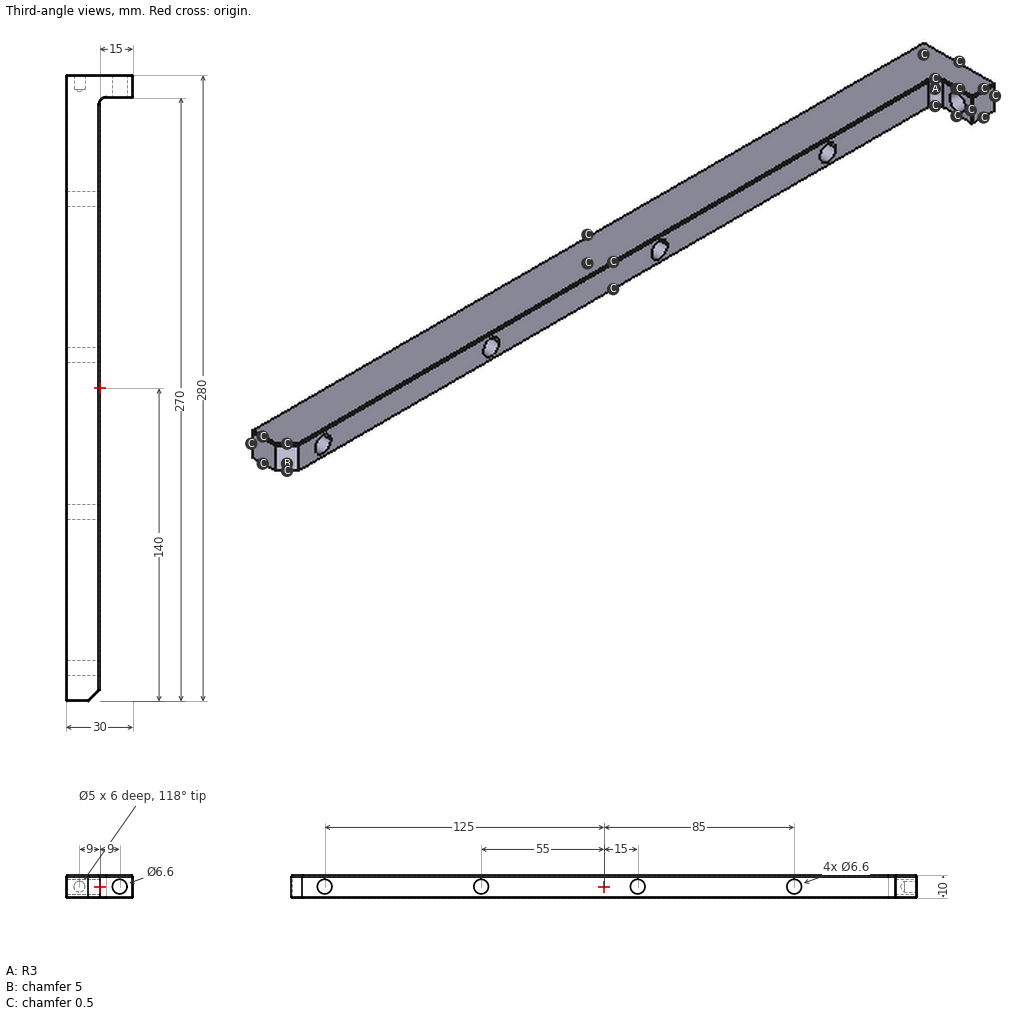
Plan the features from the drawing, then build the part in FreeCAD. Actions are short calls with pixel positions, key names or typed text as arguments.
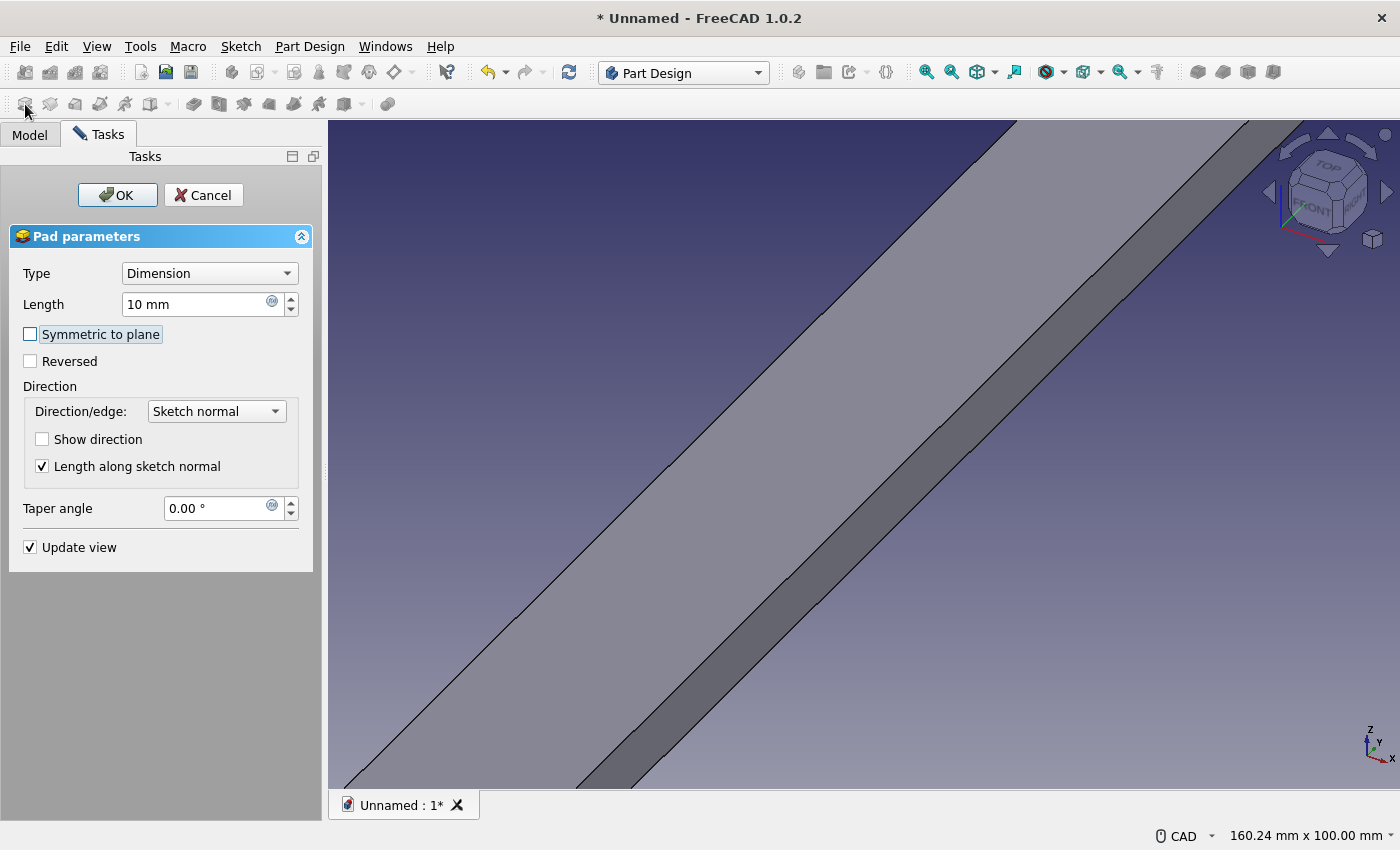
click(31, 334)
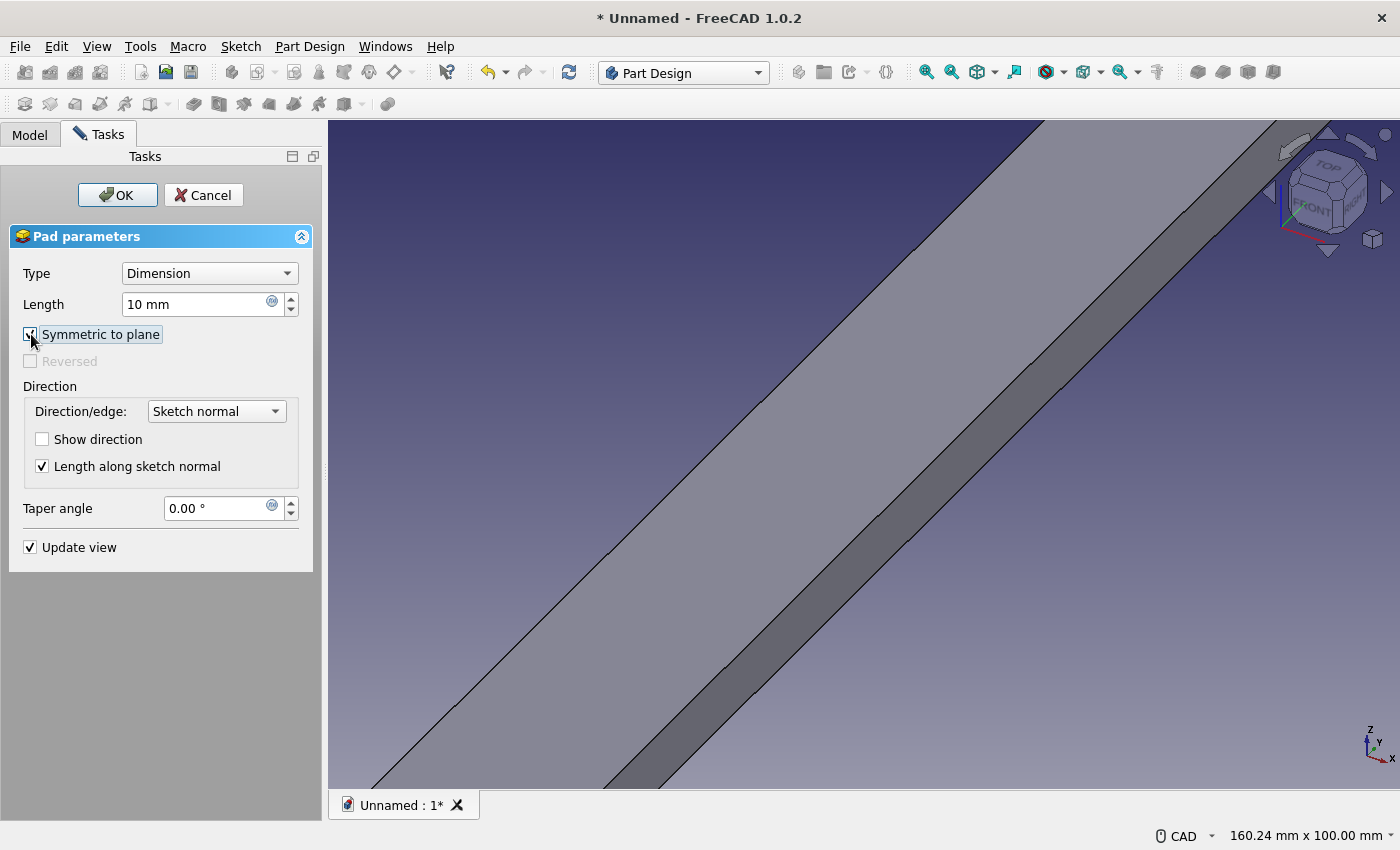
click(118, 195)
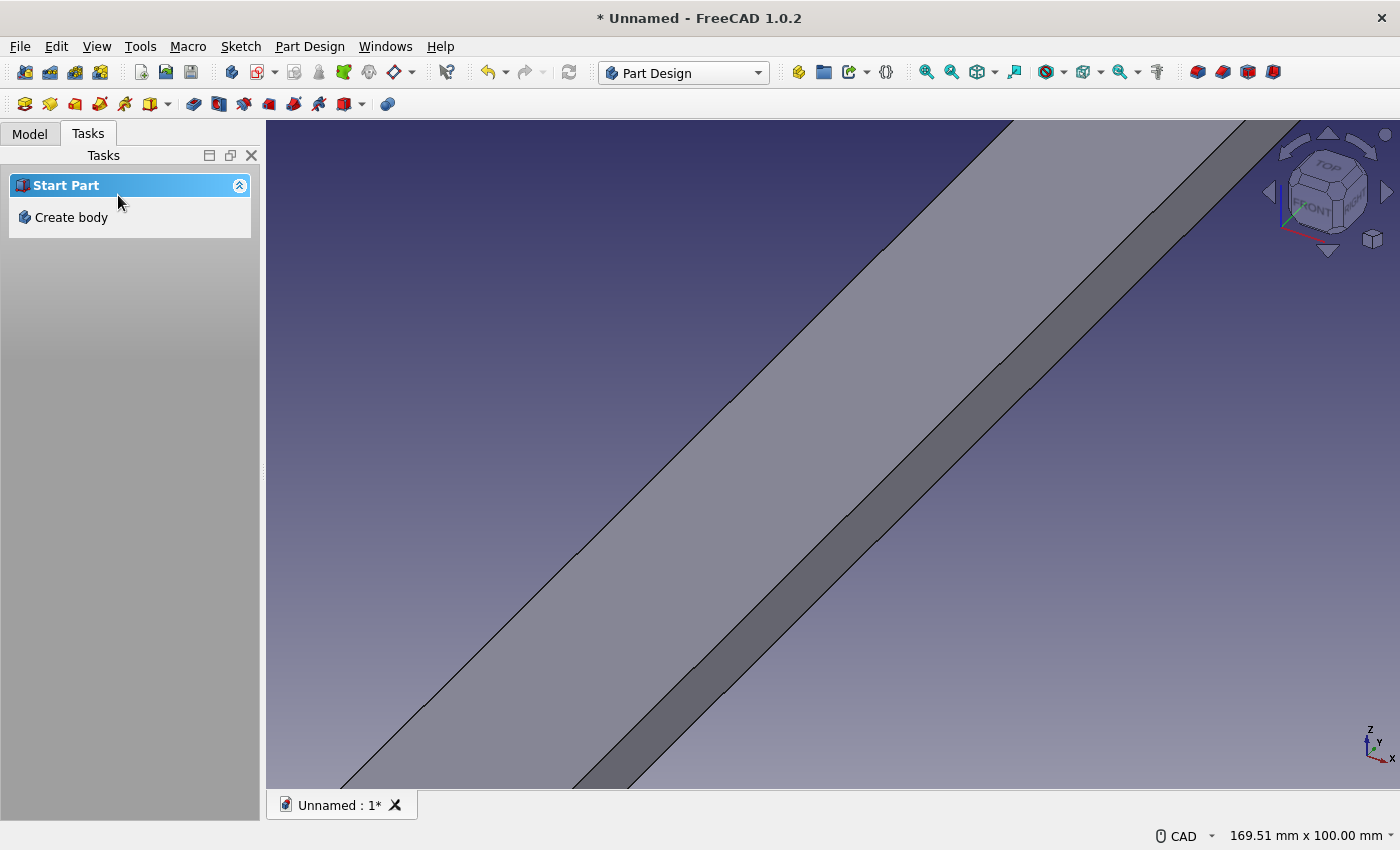
key(v)
key(f)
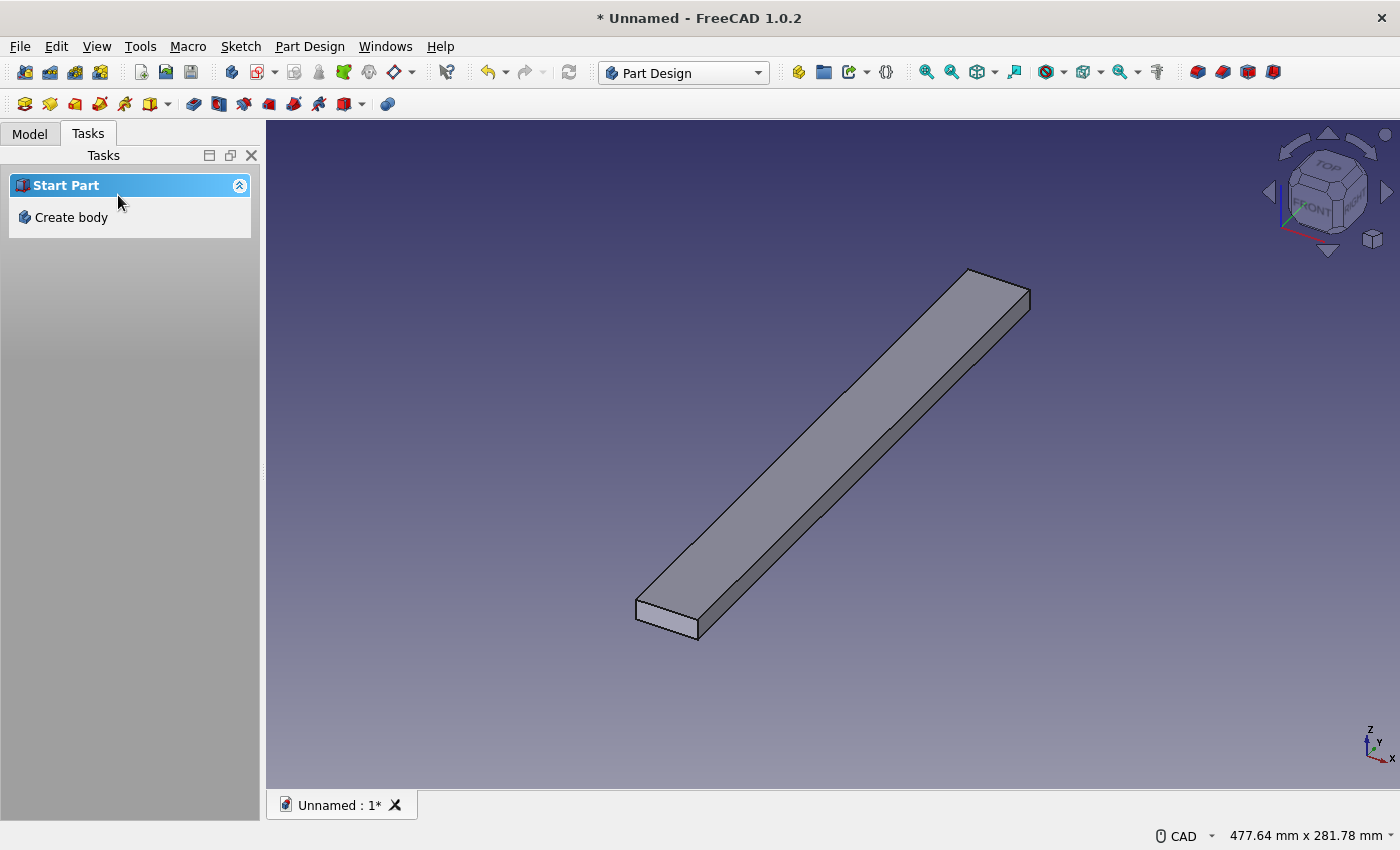
key(5)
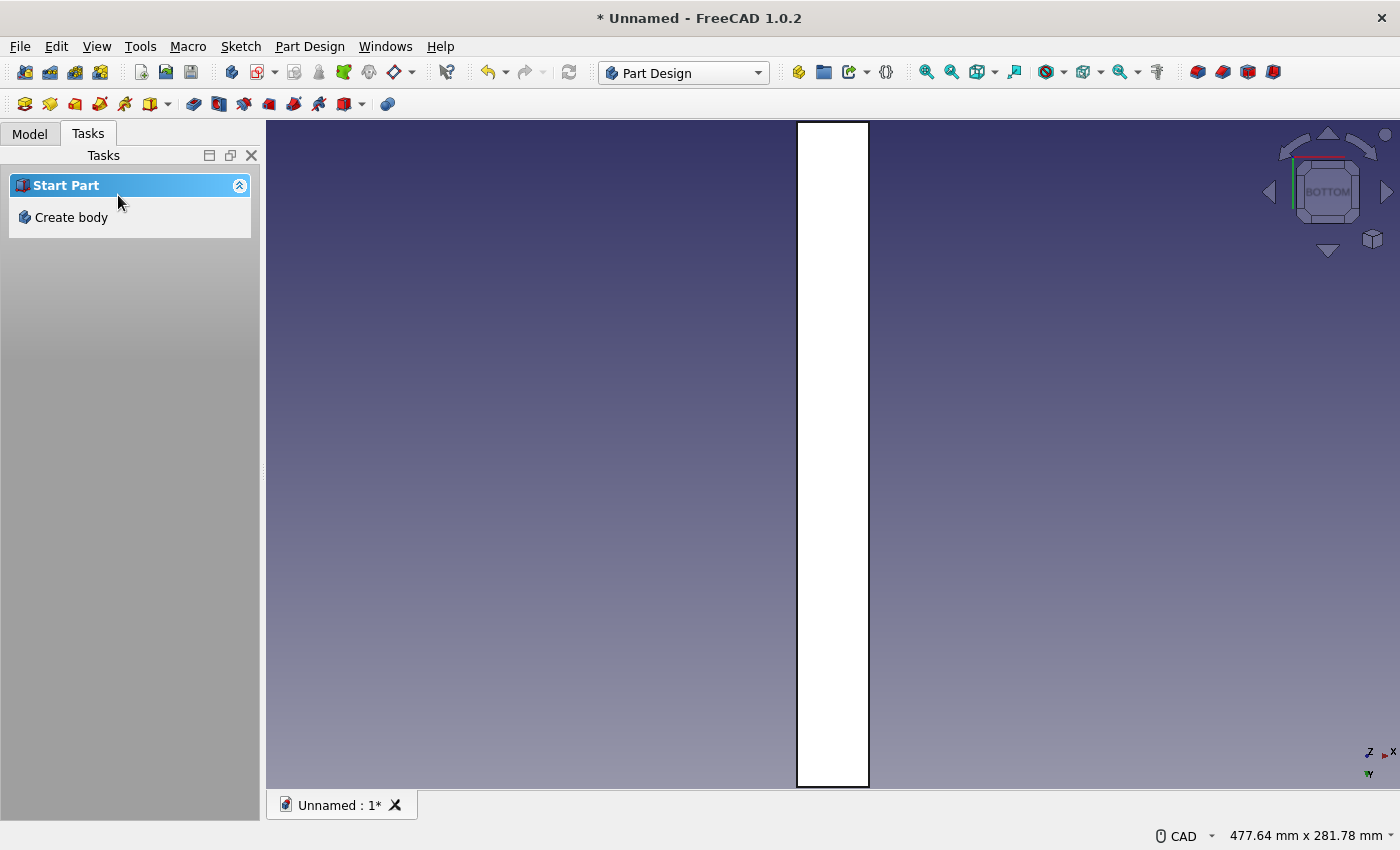
click(833, 738)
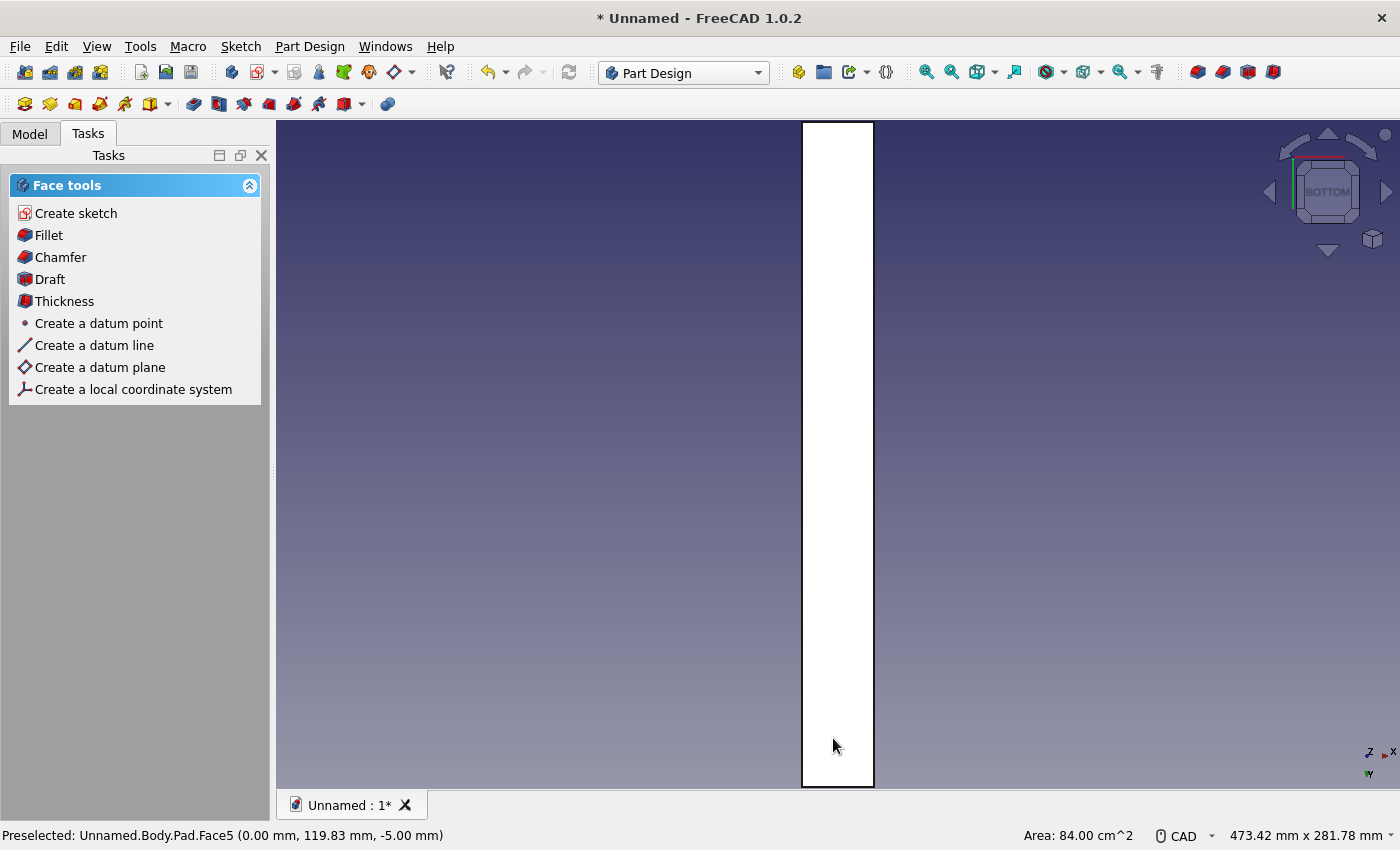
click(256, 72)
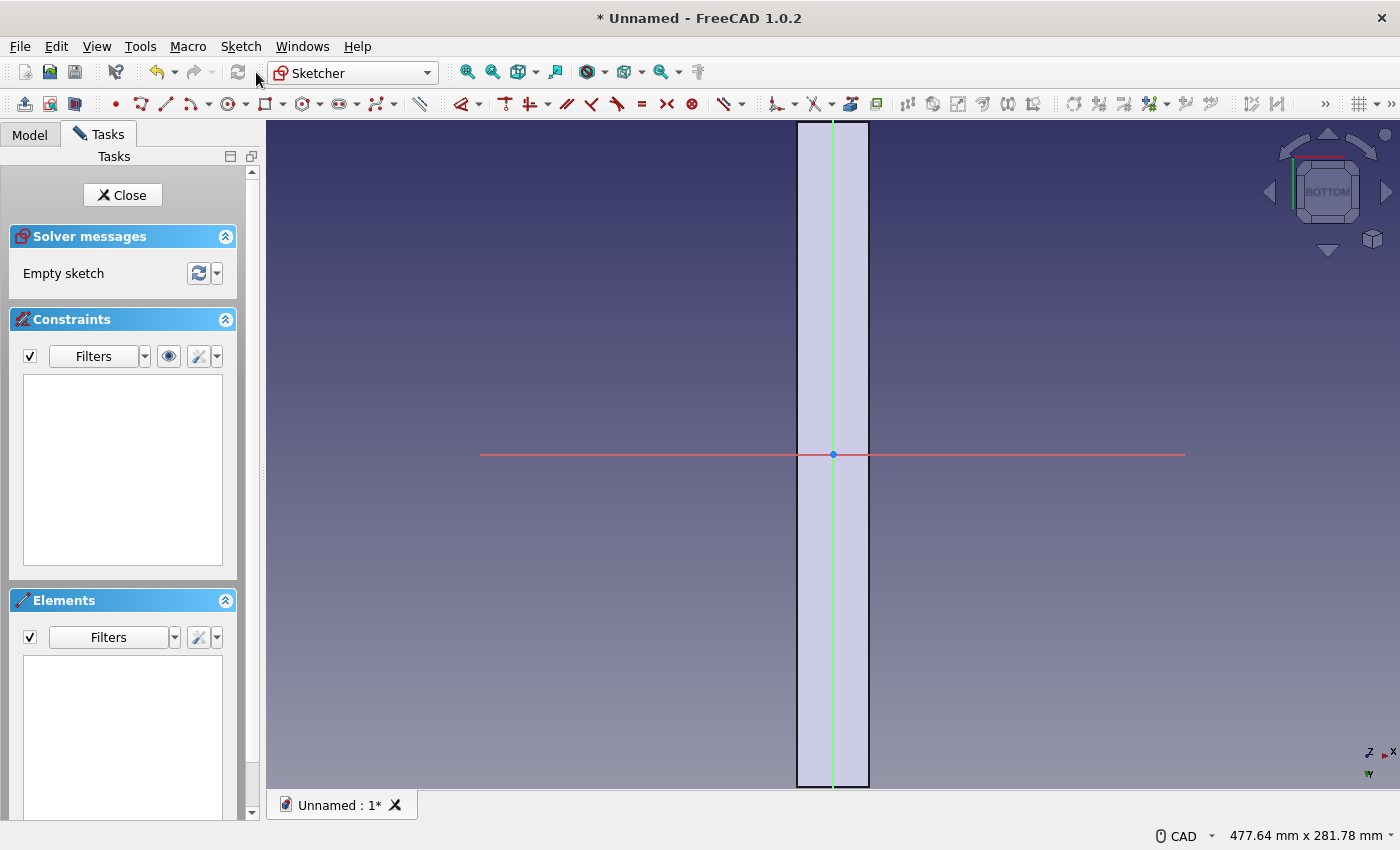
scroll(589, 479, down, 2)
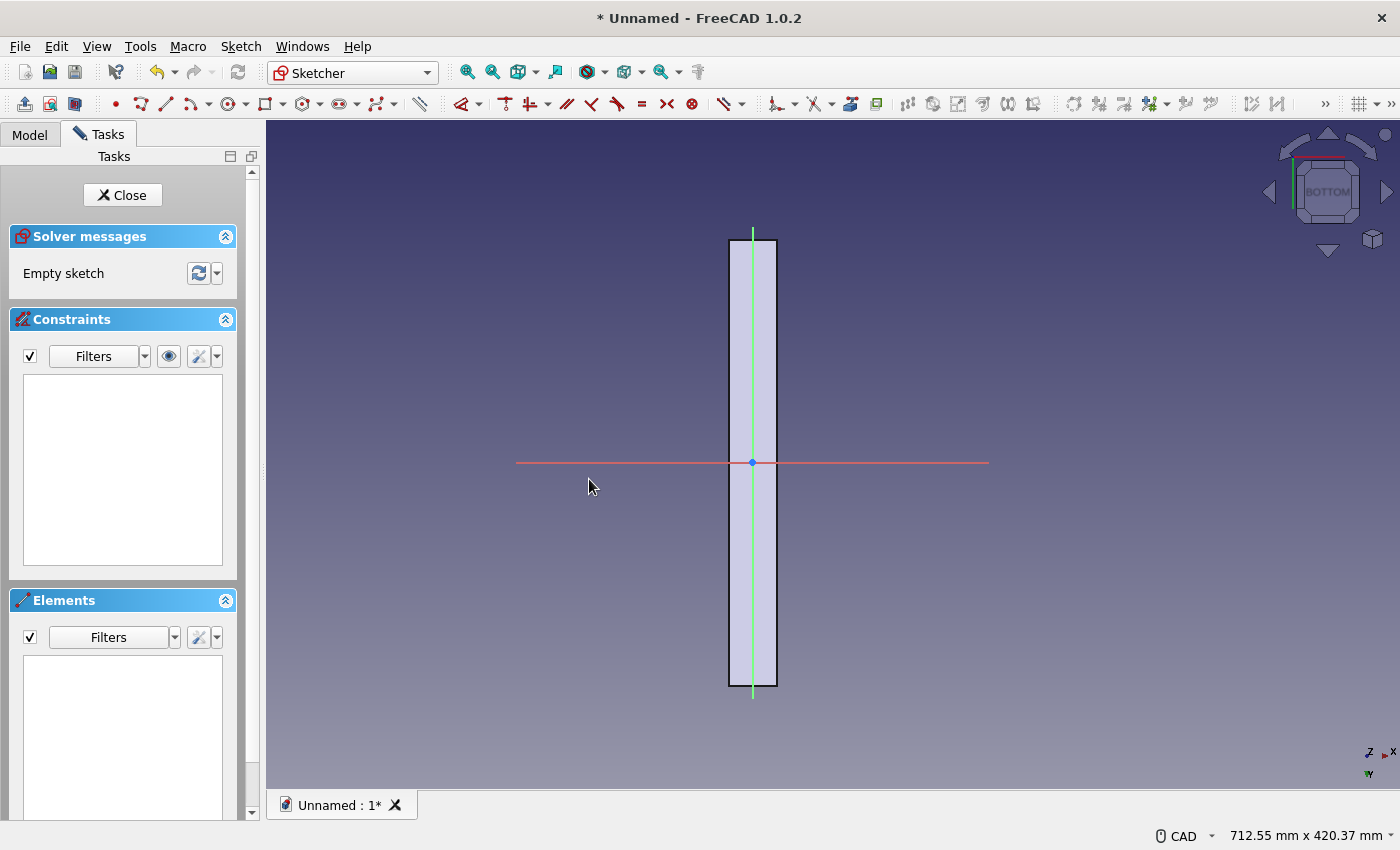
key(g)
key(r)